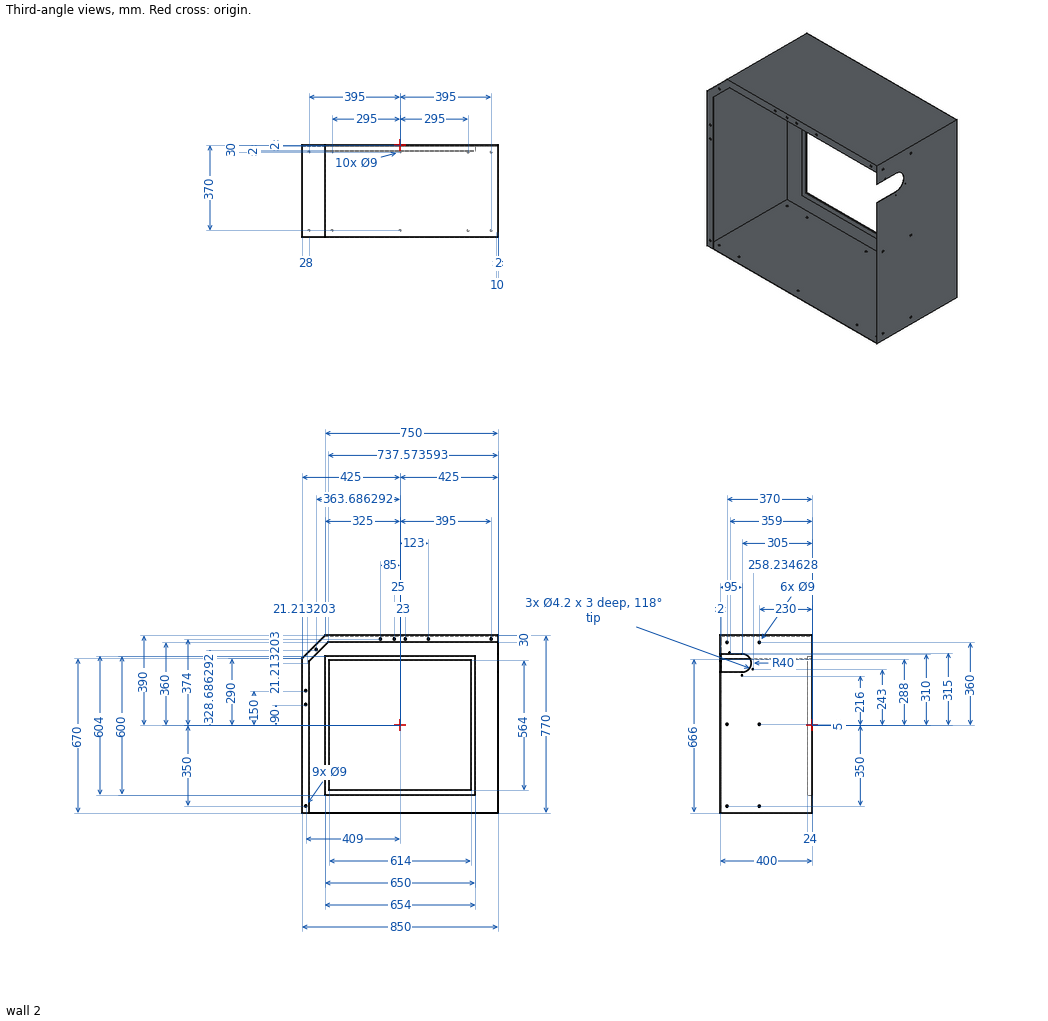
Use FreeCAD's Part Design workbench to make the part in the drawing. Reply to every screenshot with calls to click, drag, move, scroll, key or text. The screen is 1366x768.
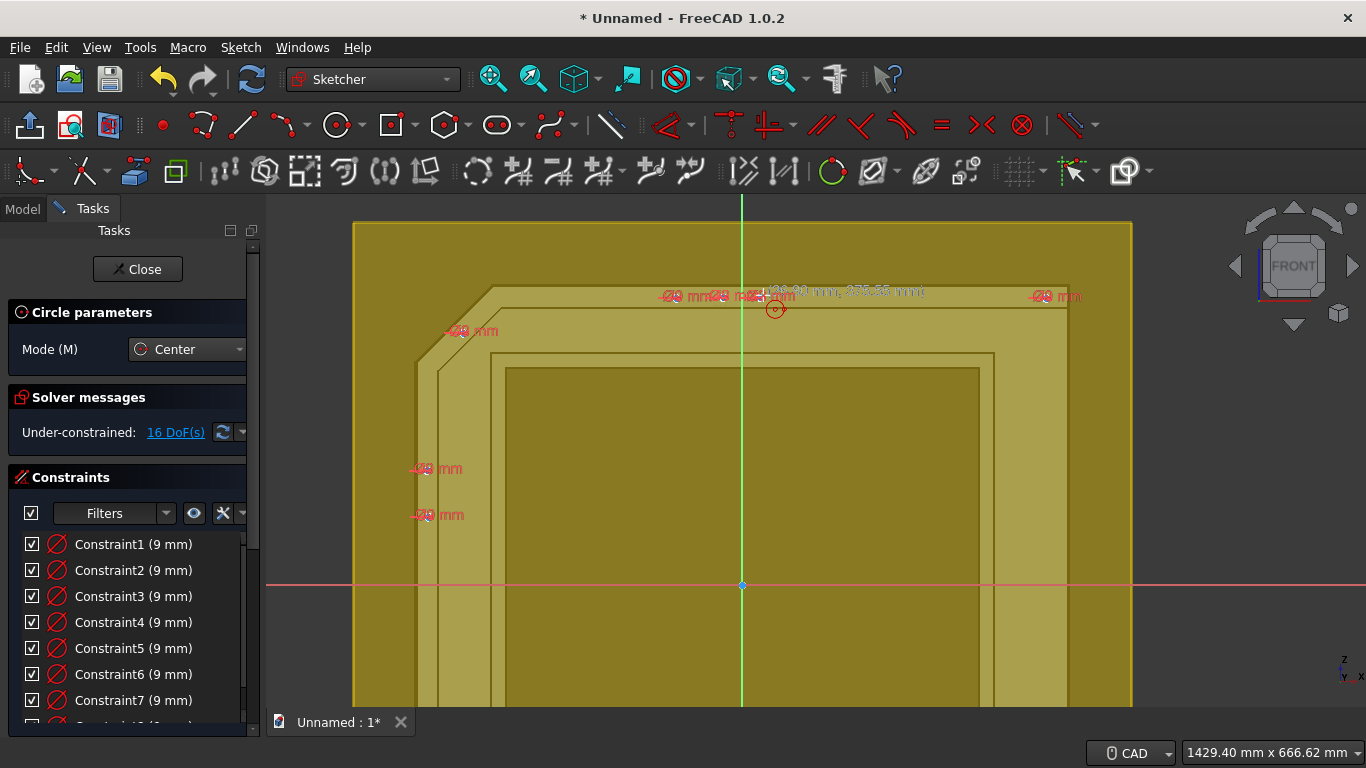
scroll(837, 297, up, 10)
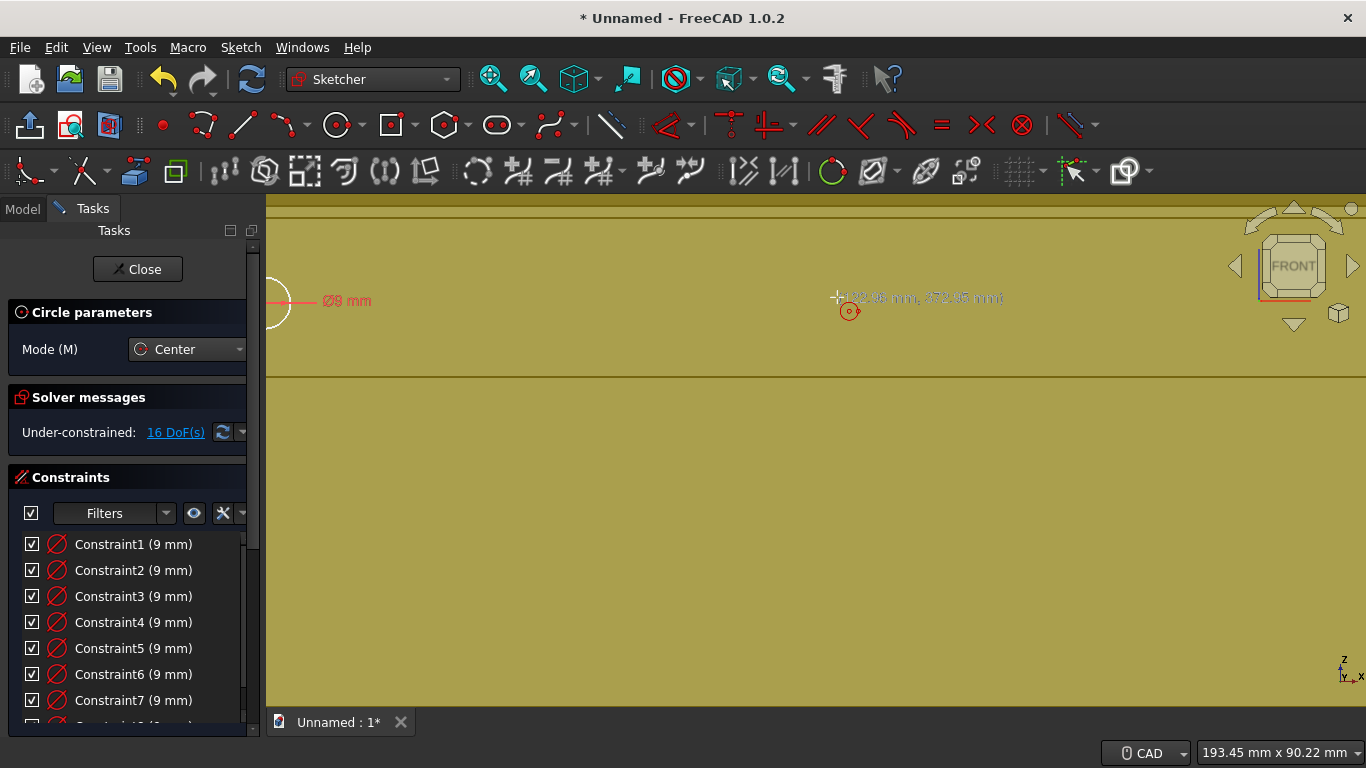
scroll(800, 298, down, 13)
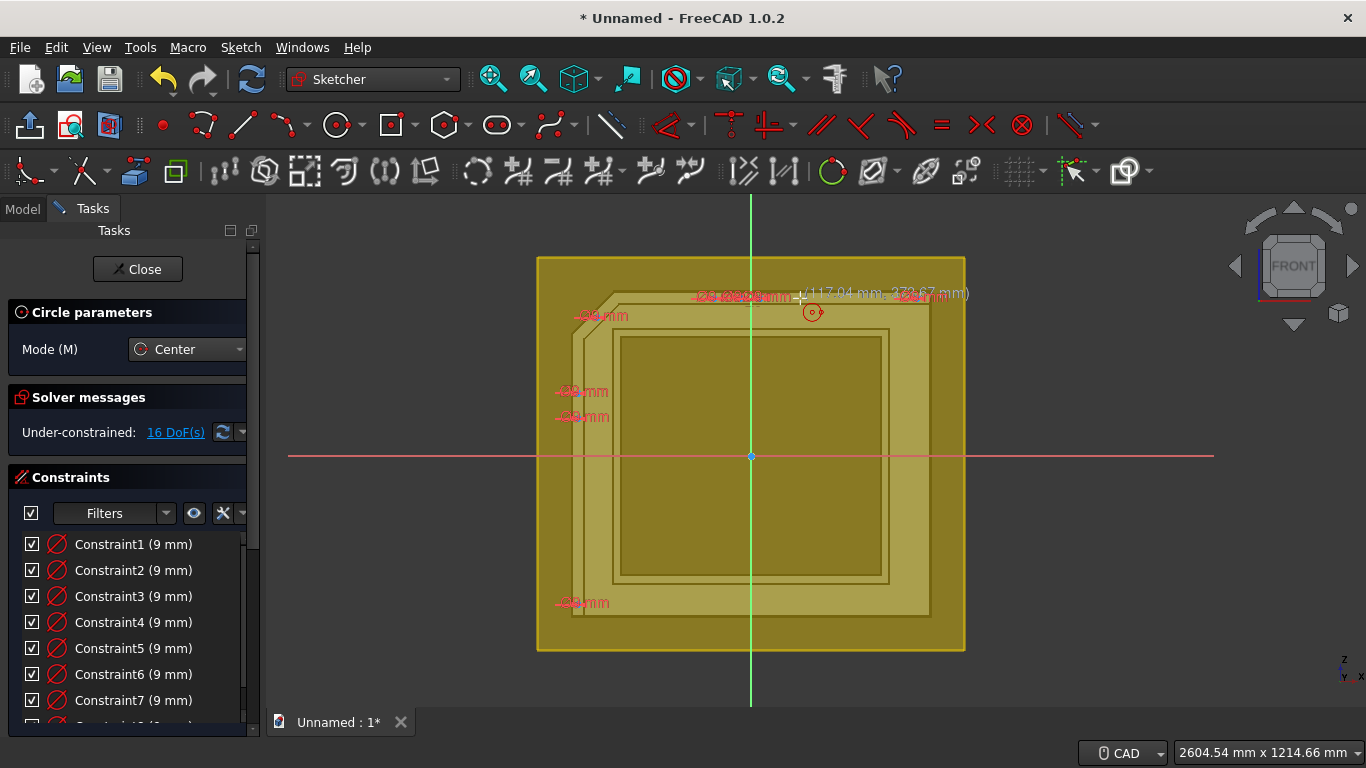
click(803, 298)
move(804, 297)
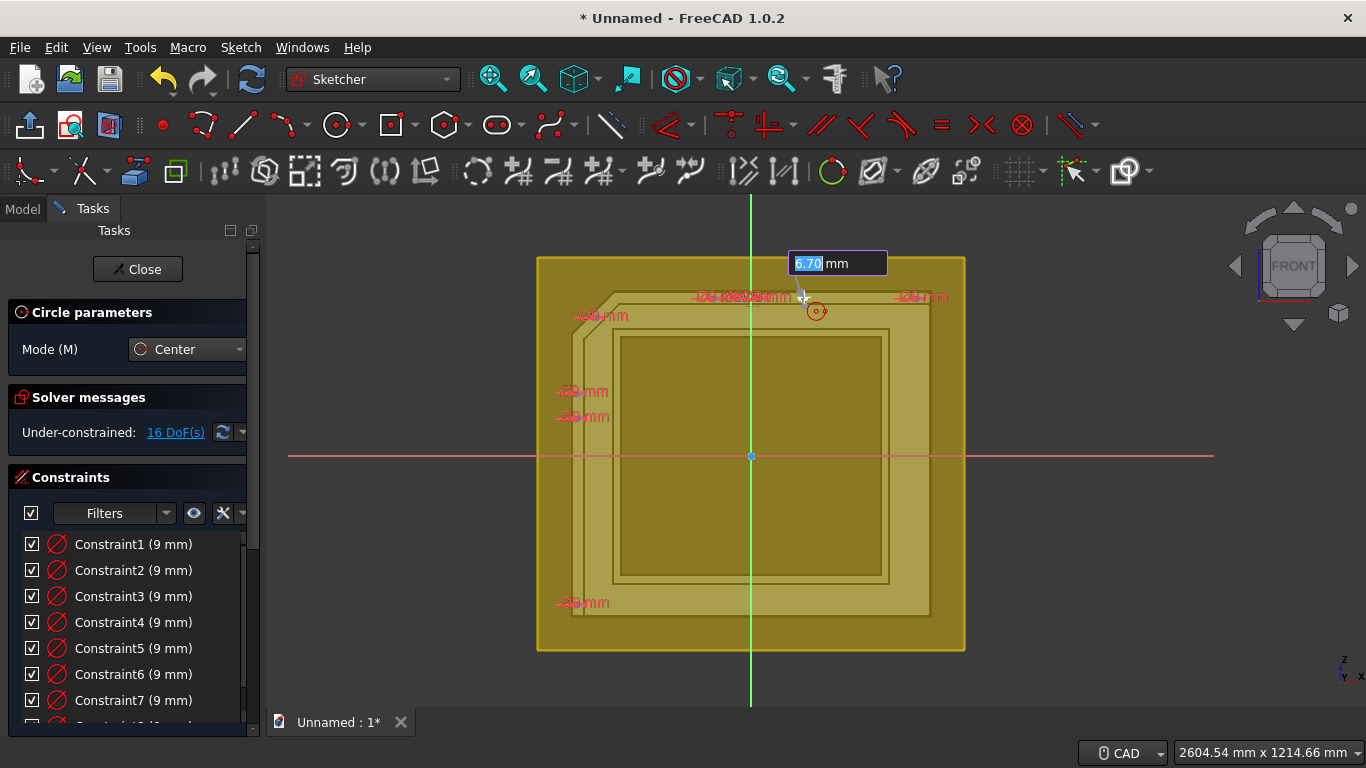
text(9)
key(Return)
key(Escape)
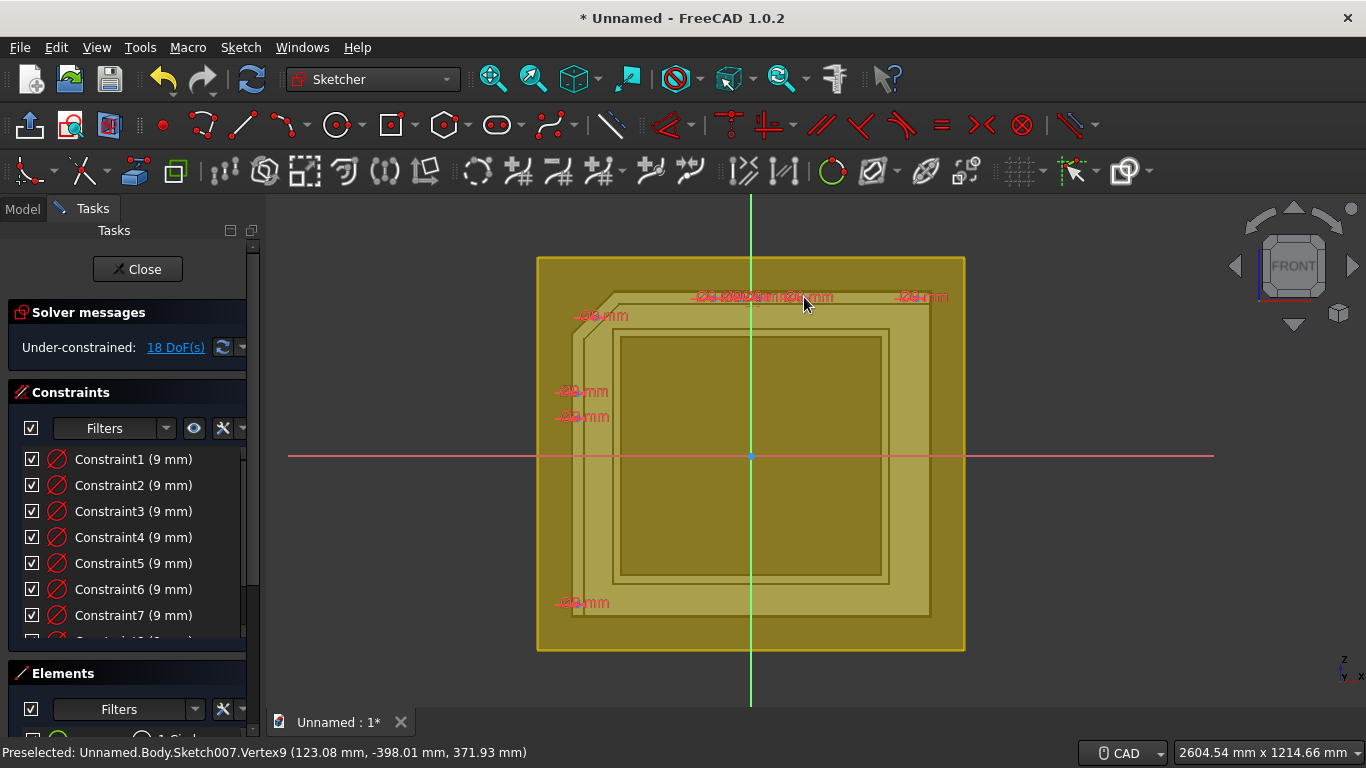
click(715, 299)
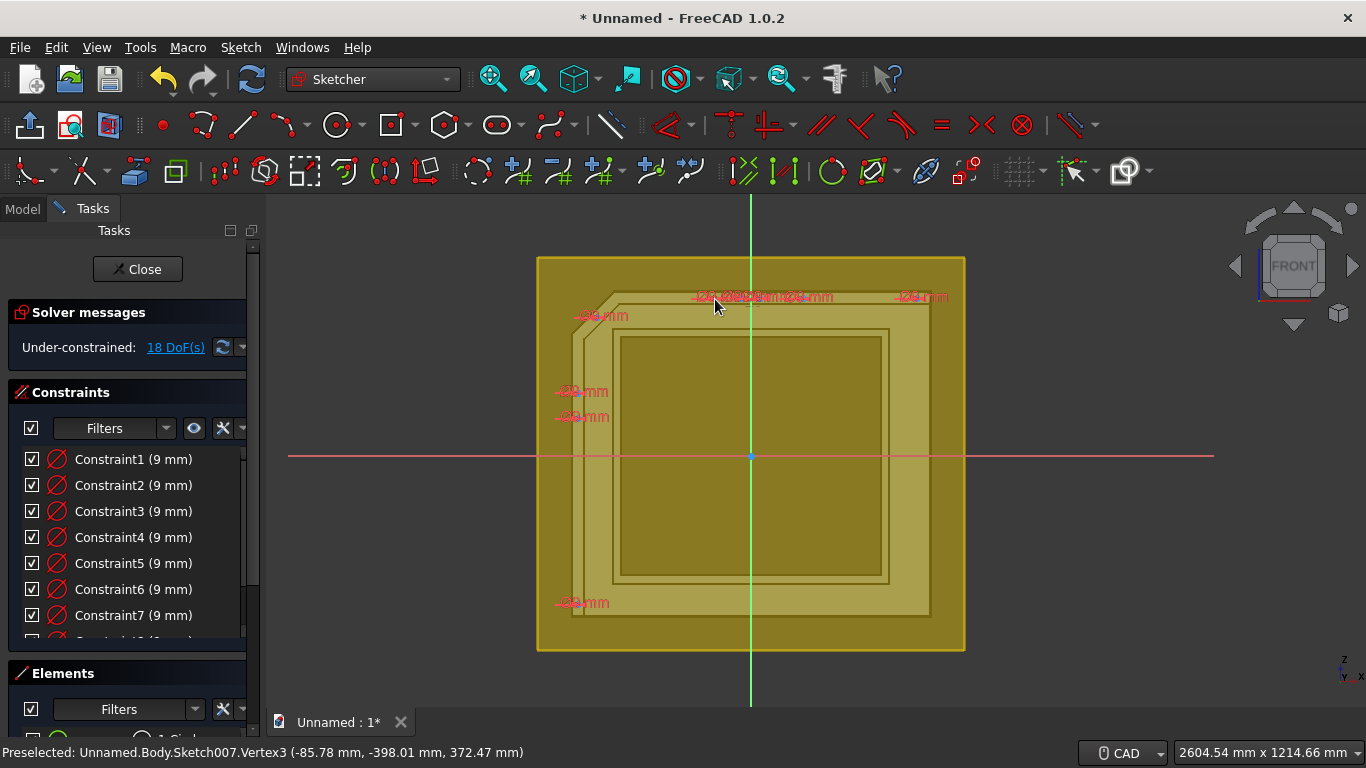
click(918, 299)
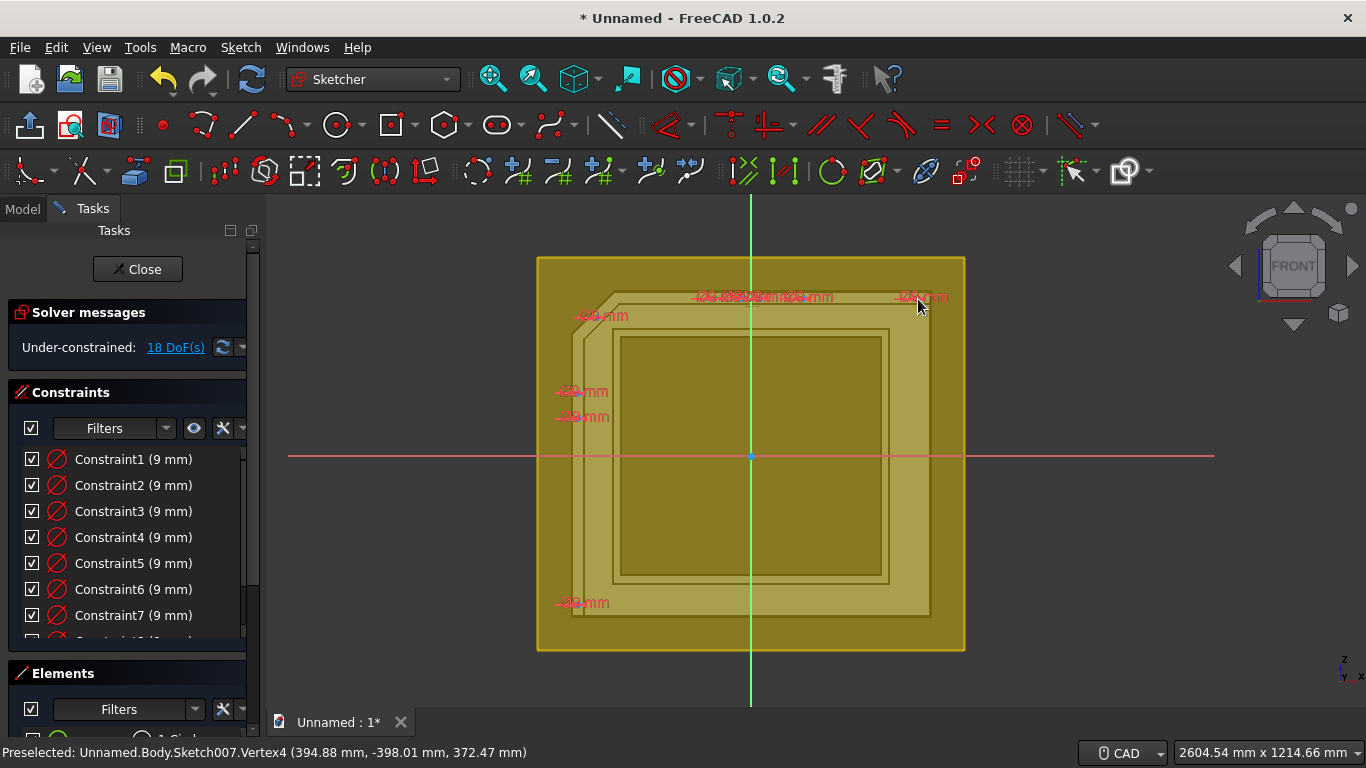
click(796, 126)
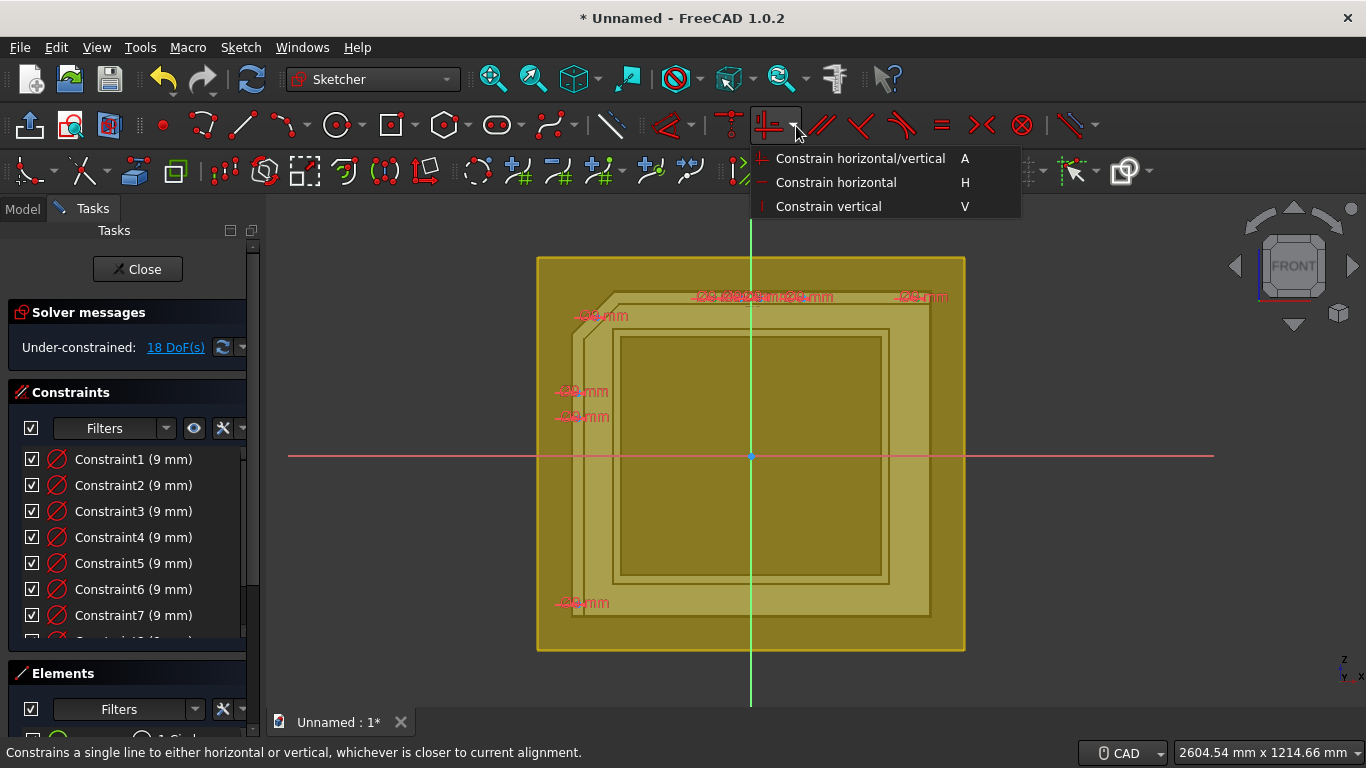
click(886, 182)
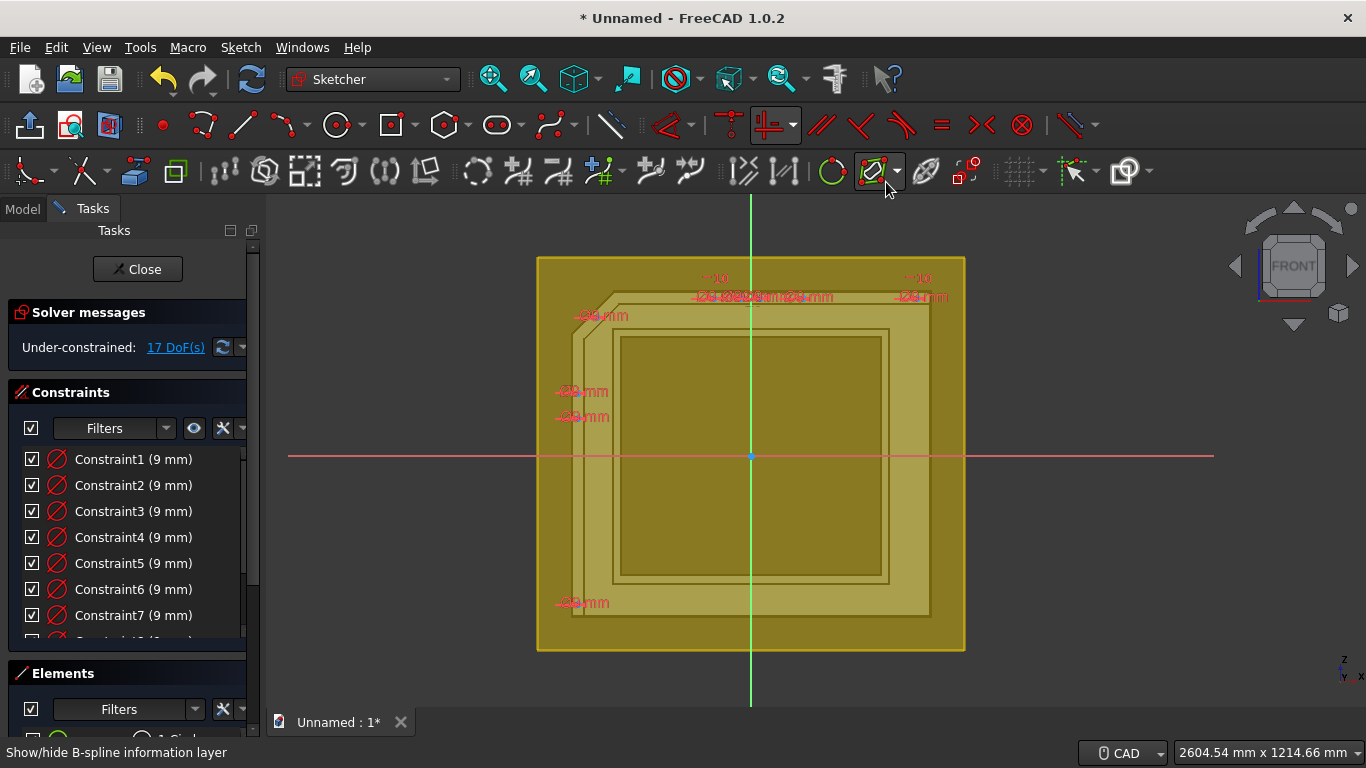
click(579, 605)